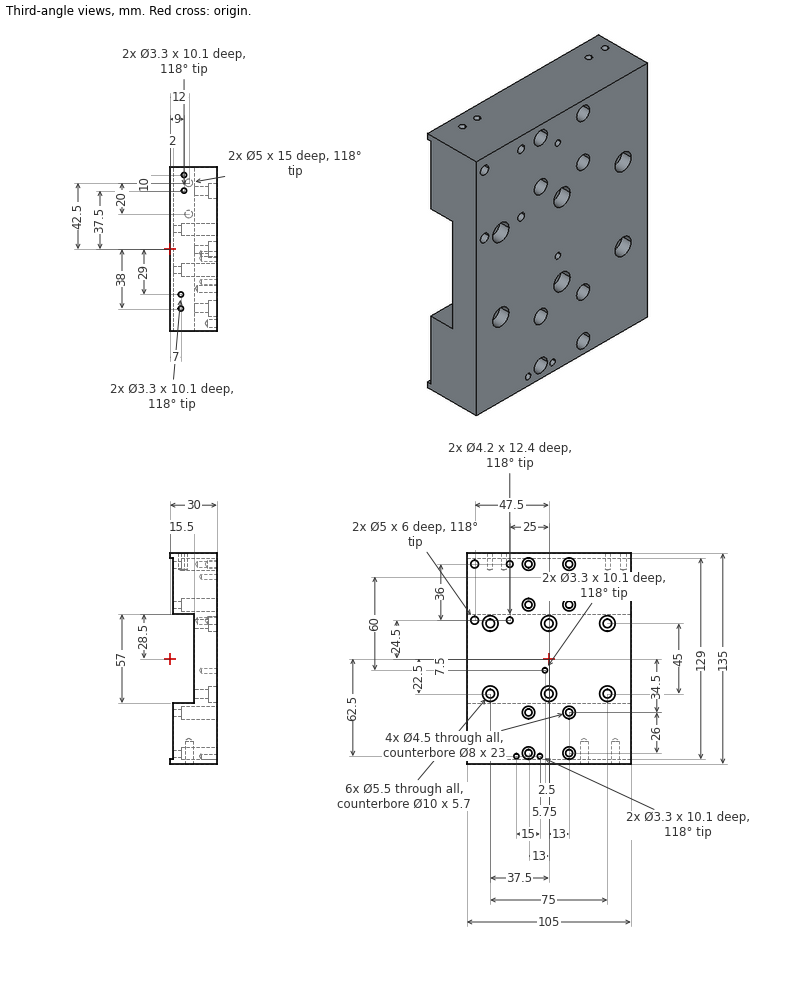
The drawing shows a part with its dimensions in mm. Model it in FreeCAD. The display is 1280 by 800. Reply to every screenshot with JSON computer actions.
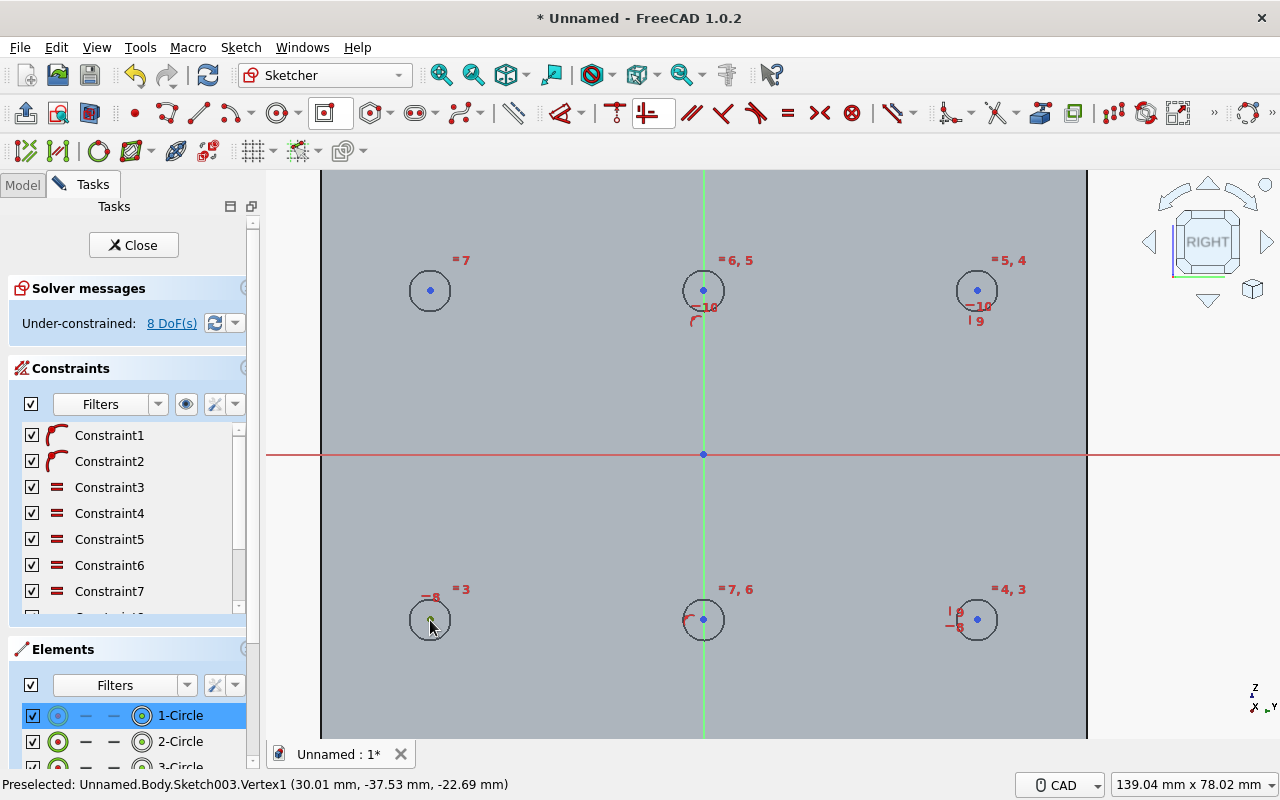
{"action": "left_click", "coordinate": [704, 620]}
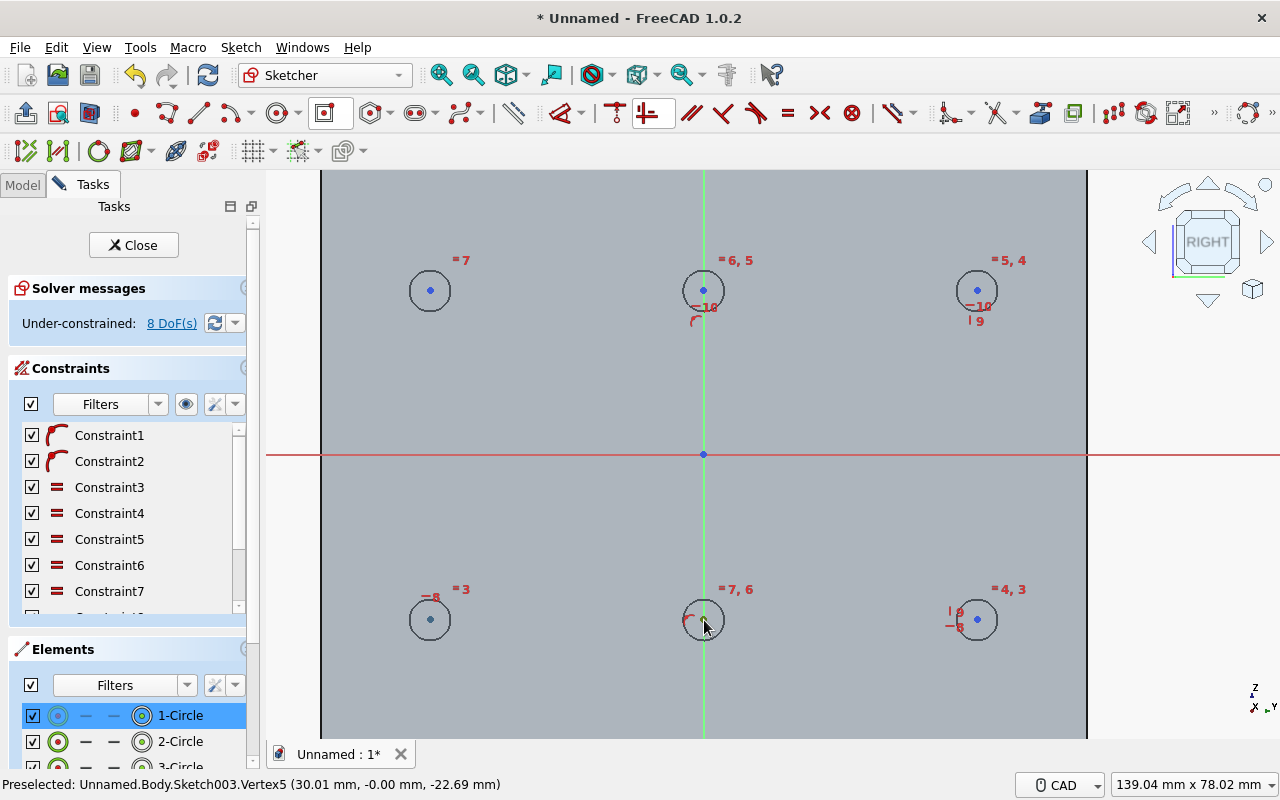
{"action": "left_click", "coordinate": [670, 114]}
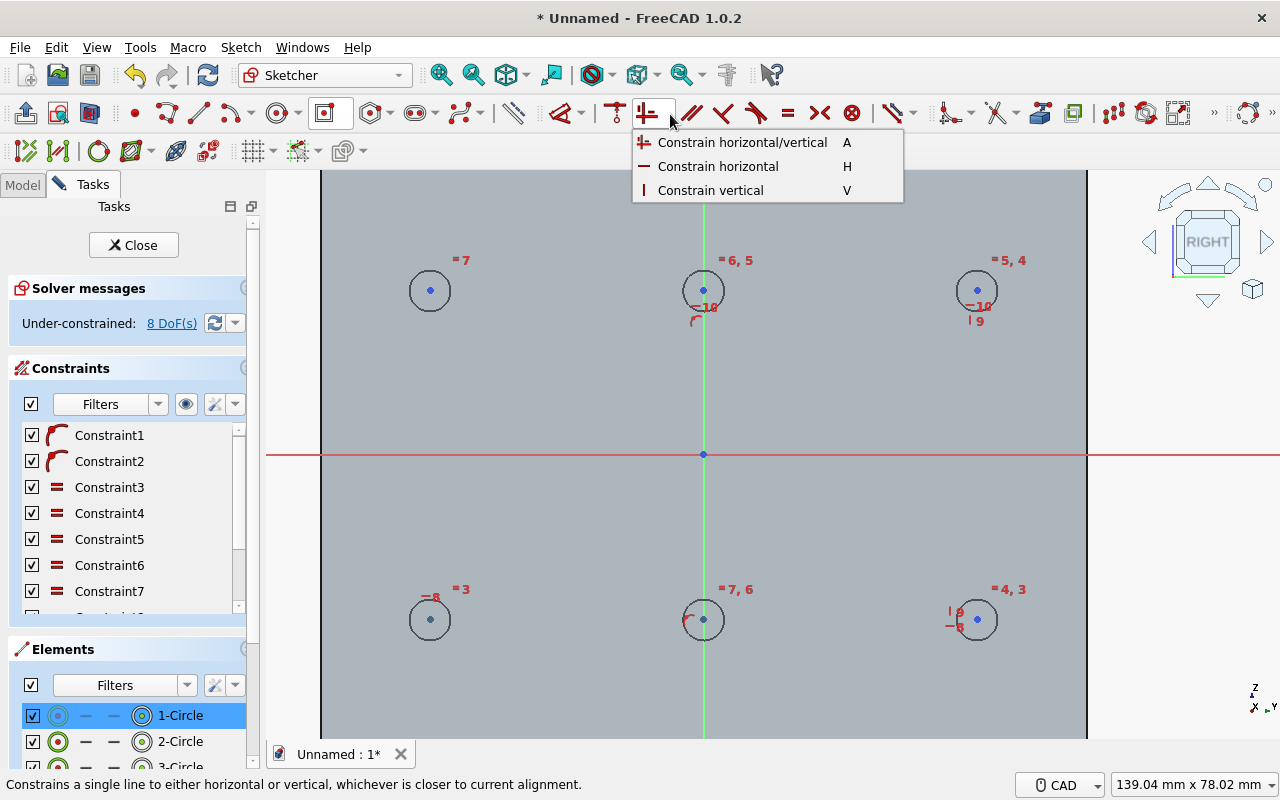
{"action": "left_click", "coordinate": [768, 166]}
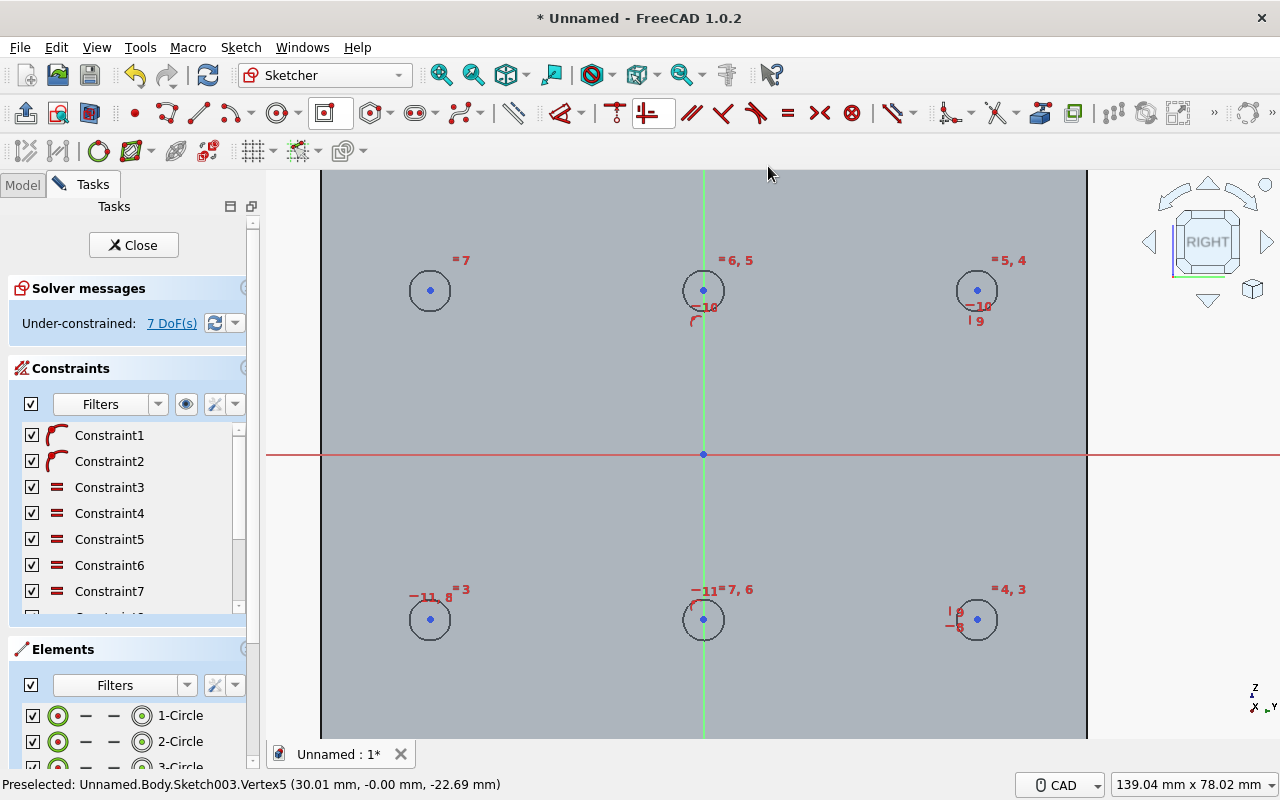
{"action": "left_click", "coordinate": [430, 620]}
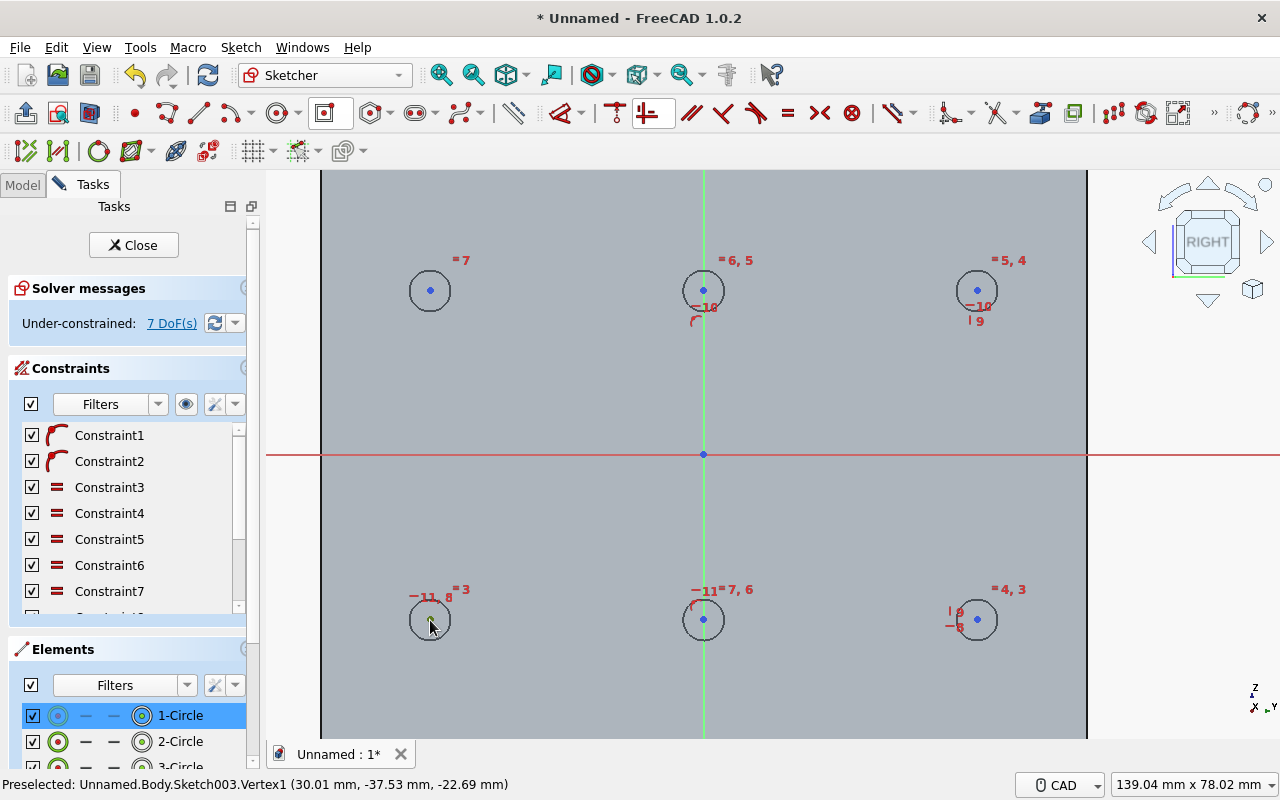
{"action": "left_click", "coordinate": [430, 291]}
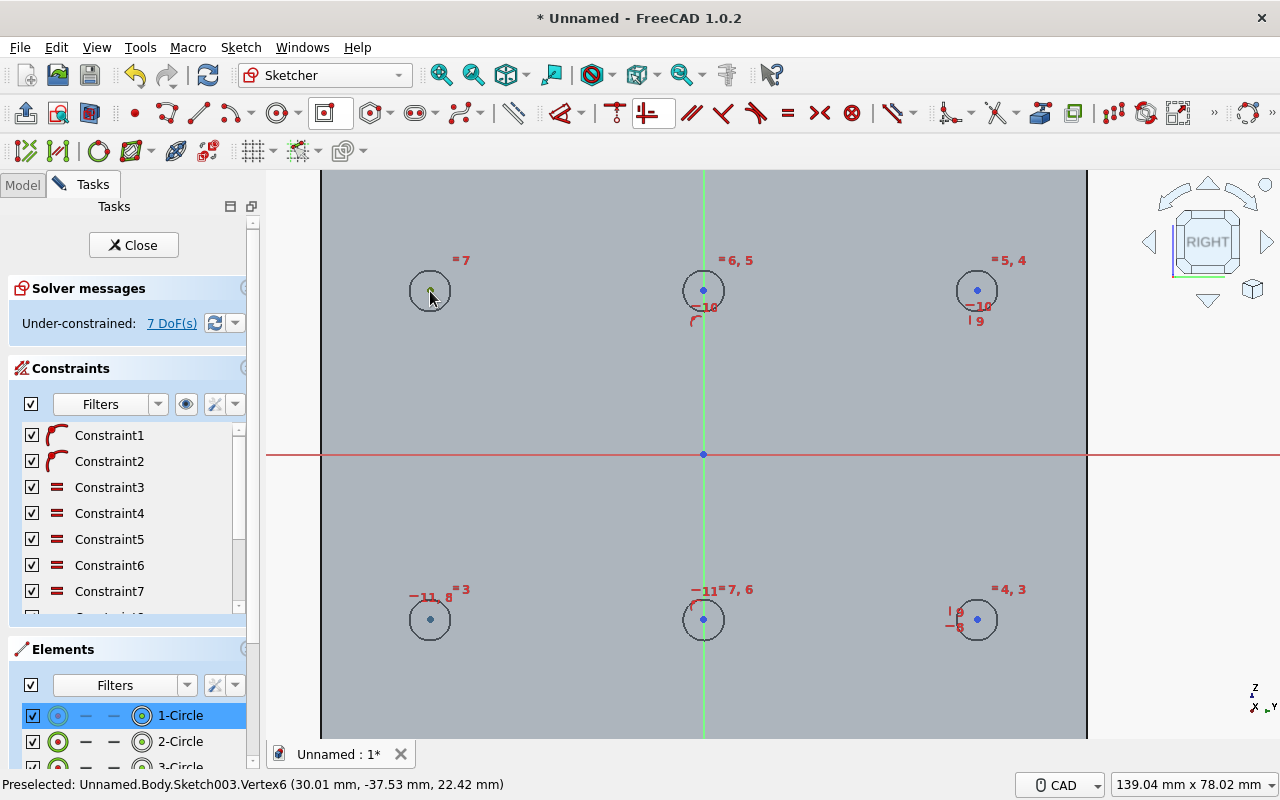
{"action": "left_click", "coordinate": [670, 114]}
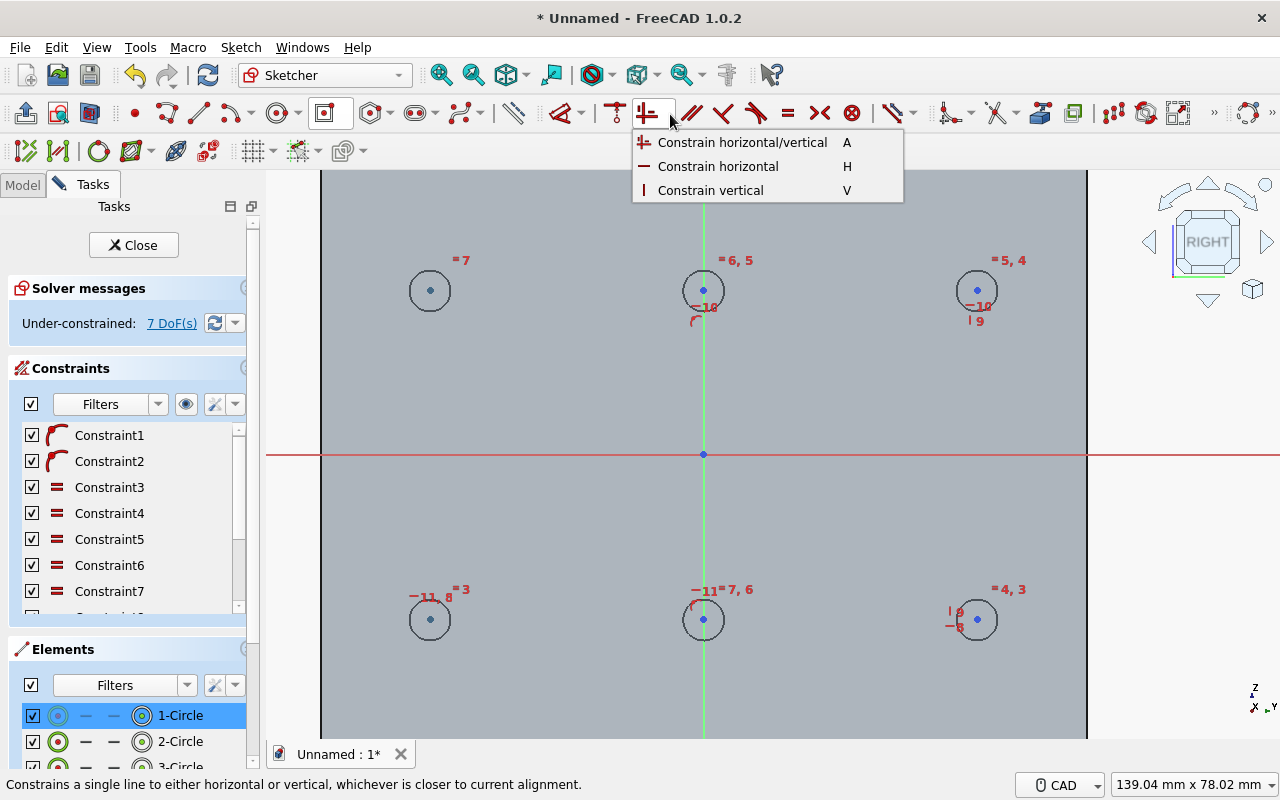
{"action": "left_click", "coordinate": [768, 190]}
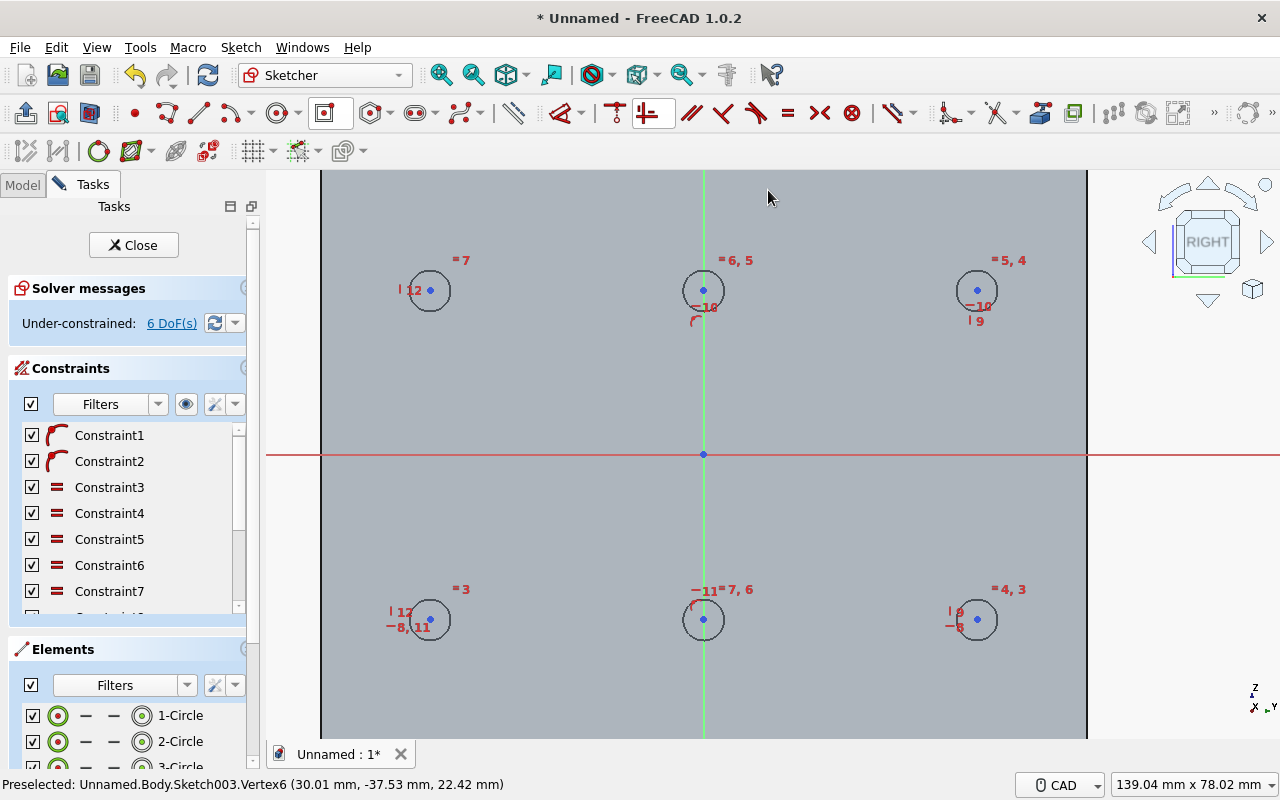
{"action": "left_click", "coordinate": [704, 291]}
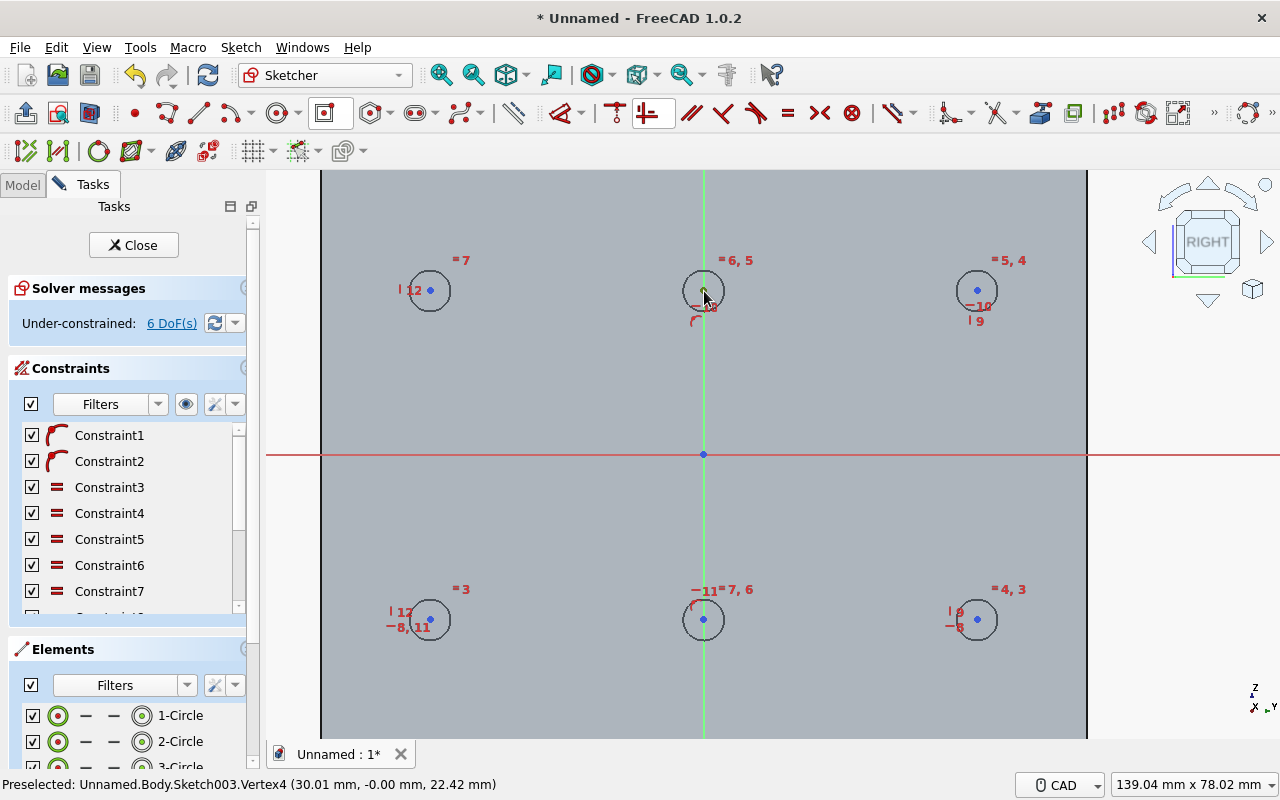
{"action": "left_click", "coordinate": [430, 291]}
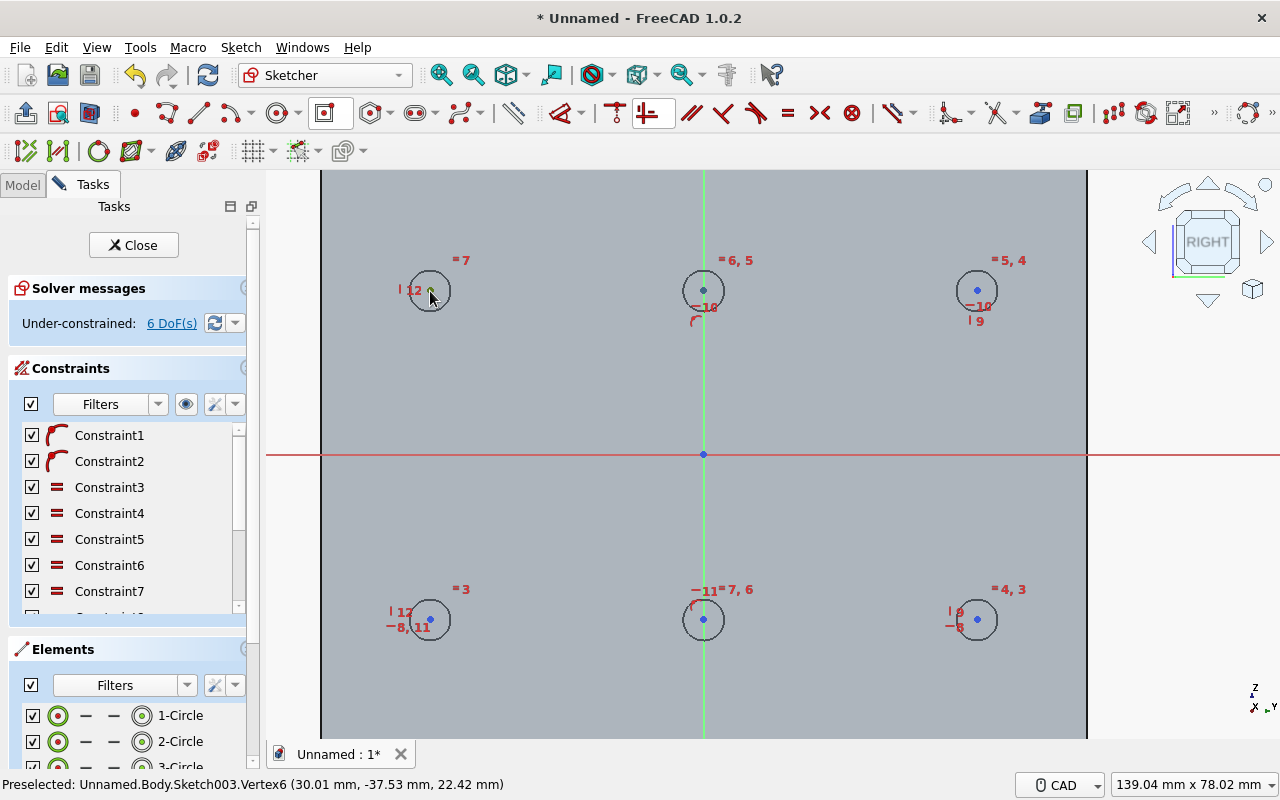
{"action": "left_click", "coordinate": [670, 114]}